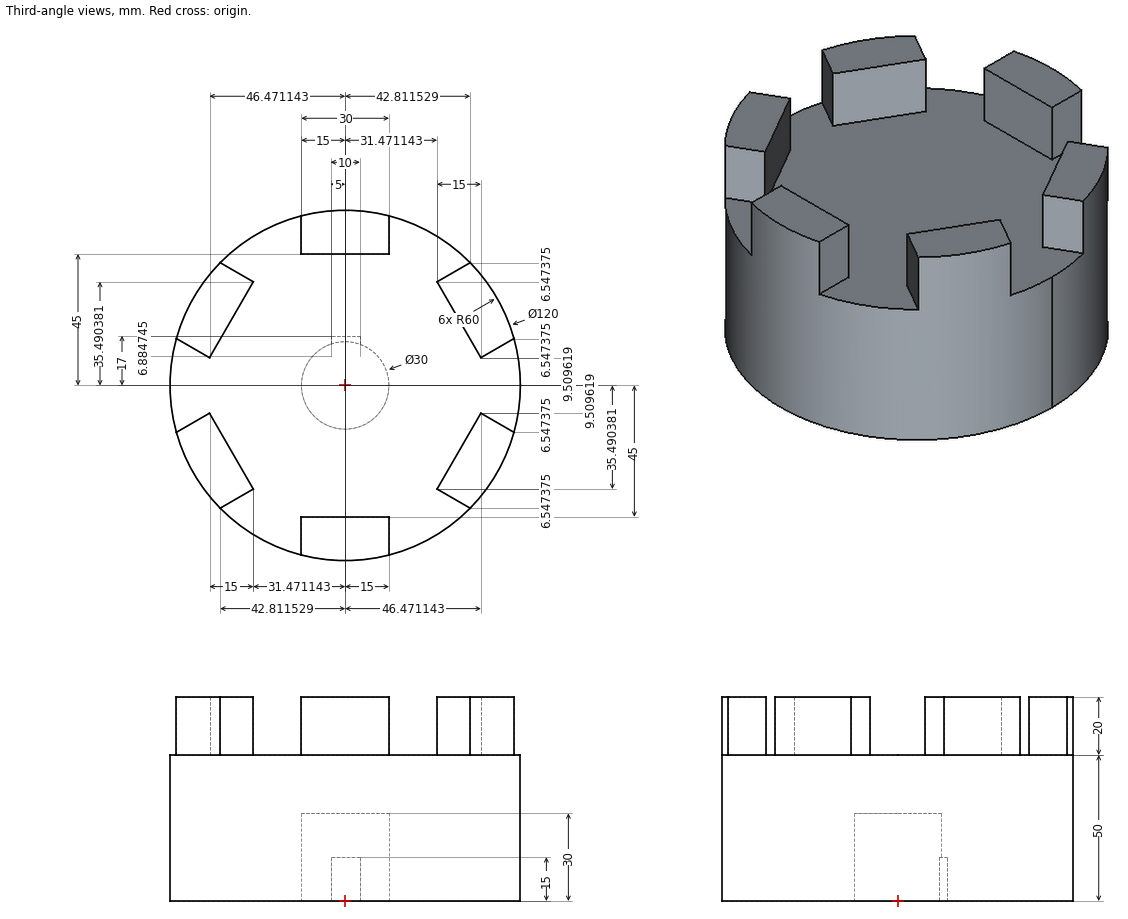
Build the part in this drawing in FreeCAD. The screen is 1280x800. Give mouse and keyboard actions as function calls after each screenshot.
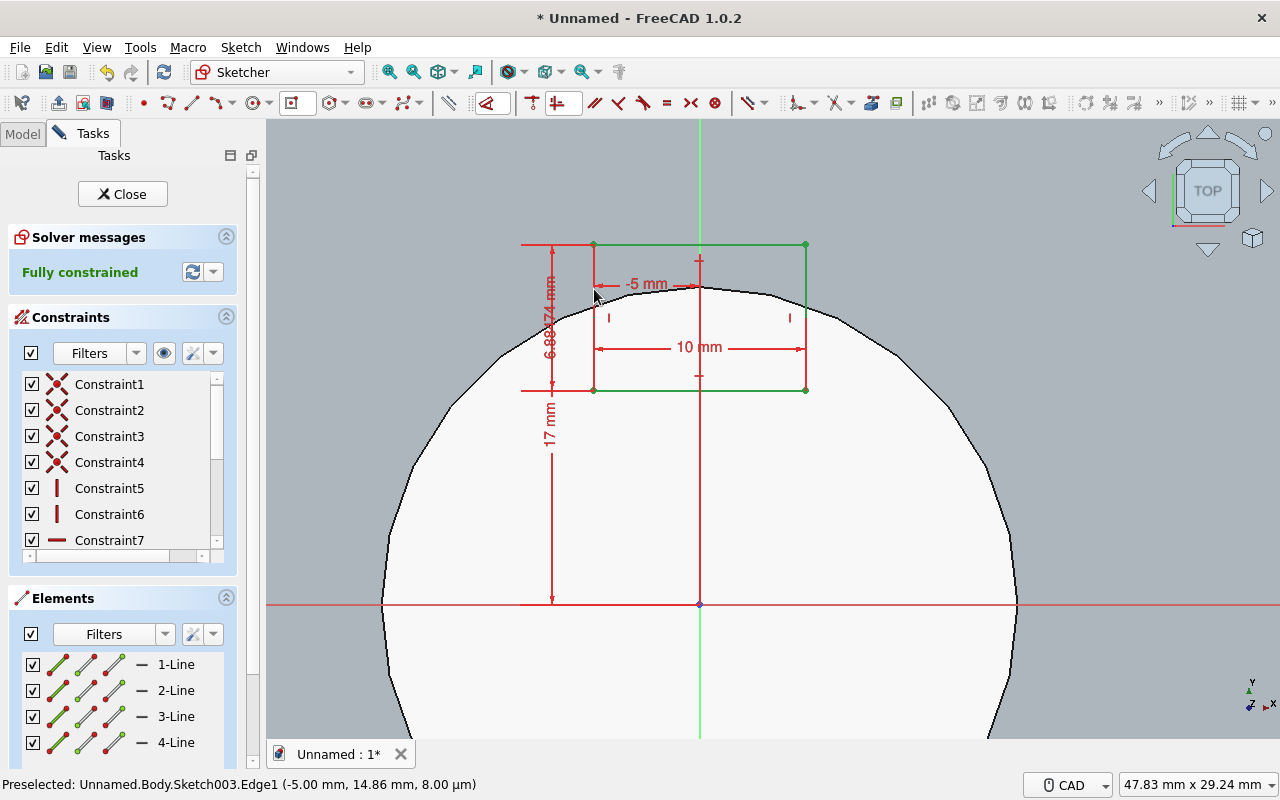
click(123, 194)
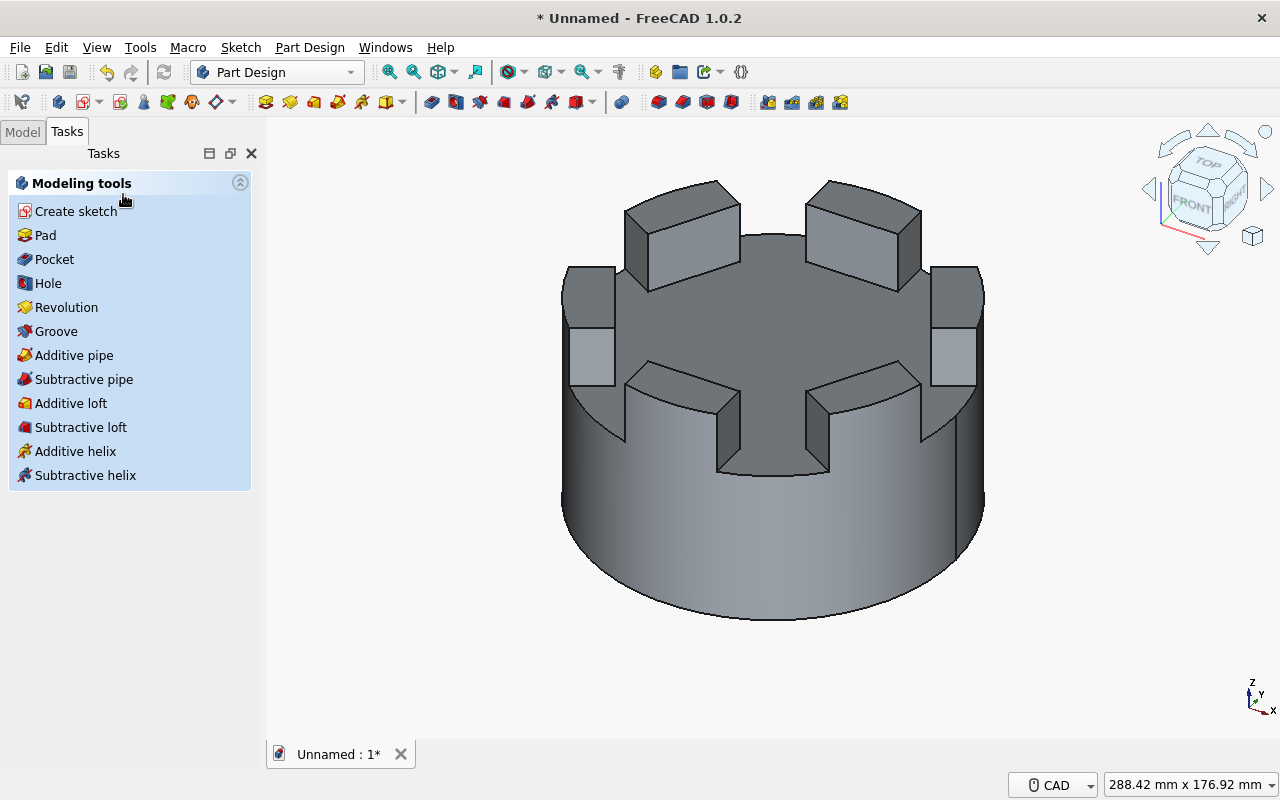
click(432, 102)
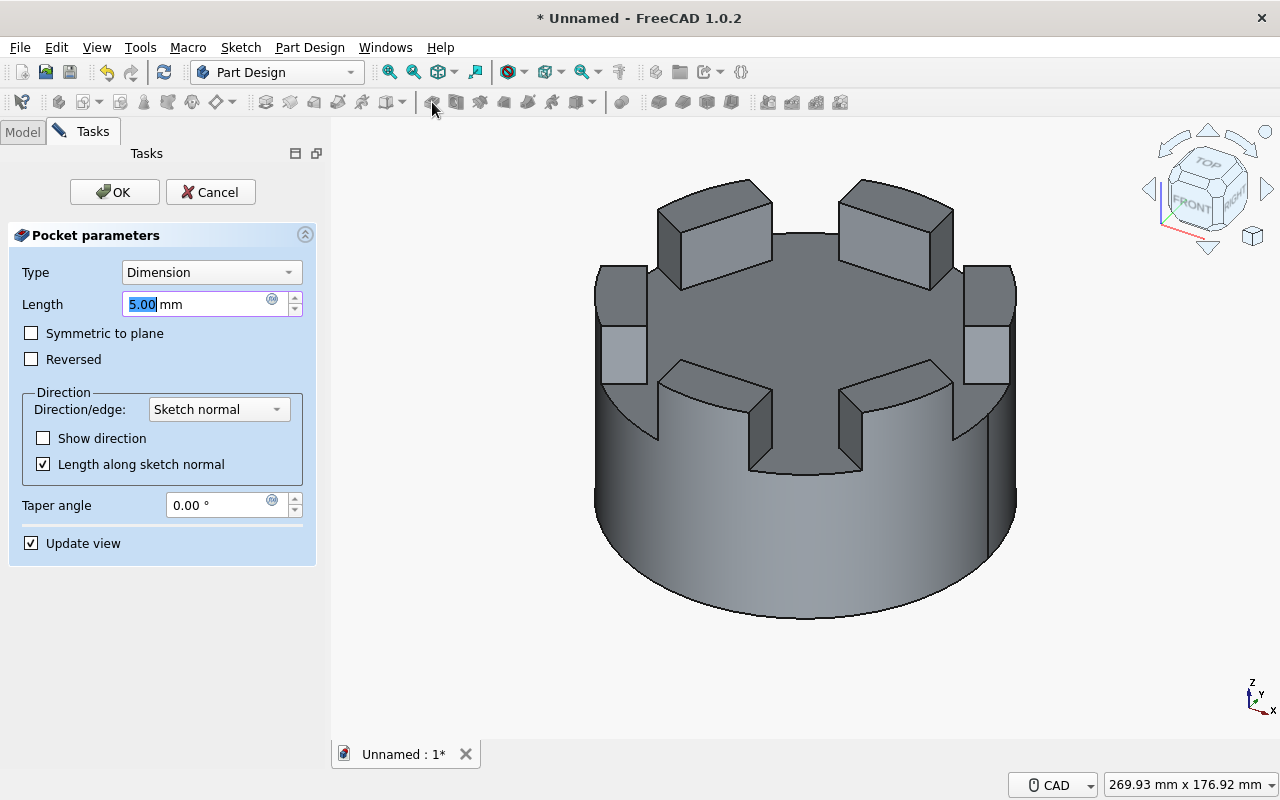
text(15)
key(Tab)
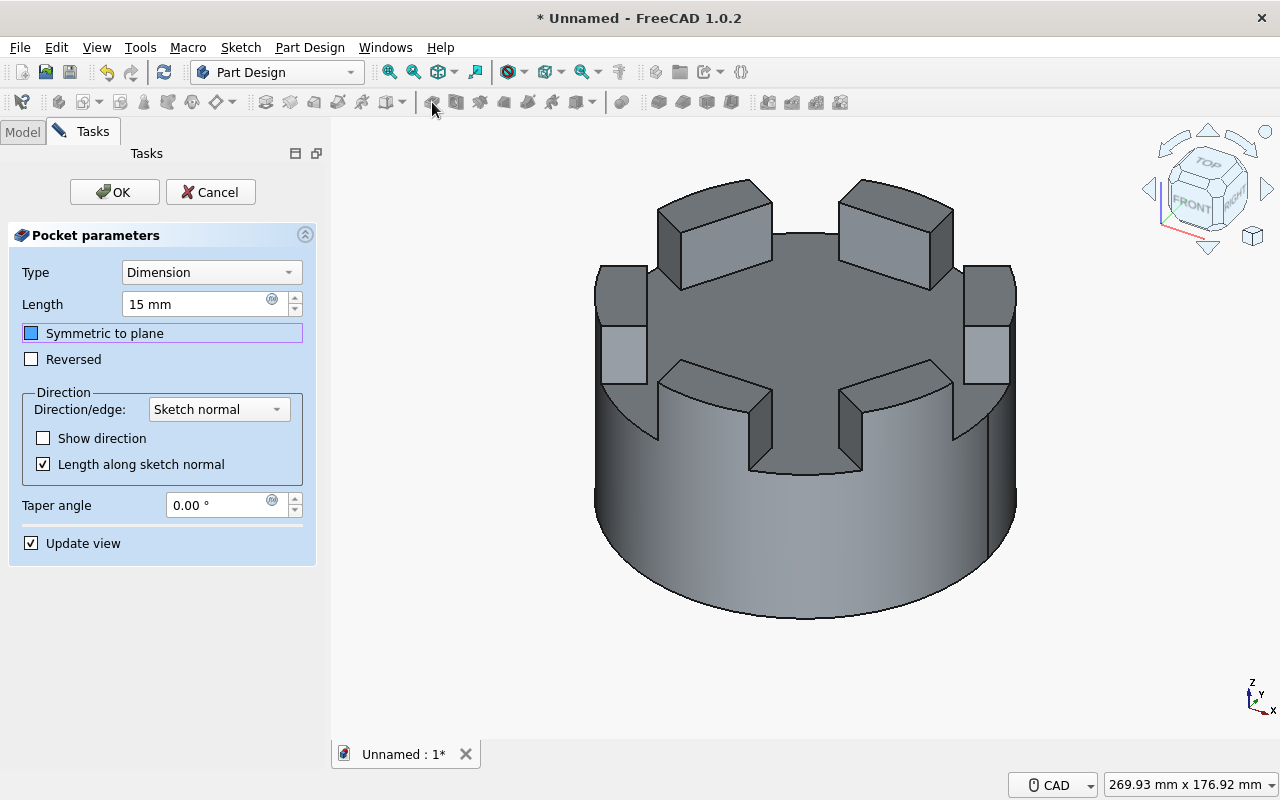
click(30, 359)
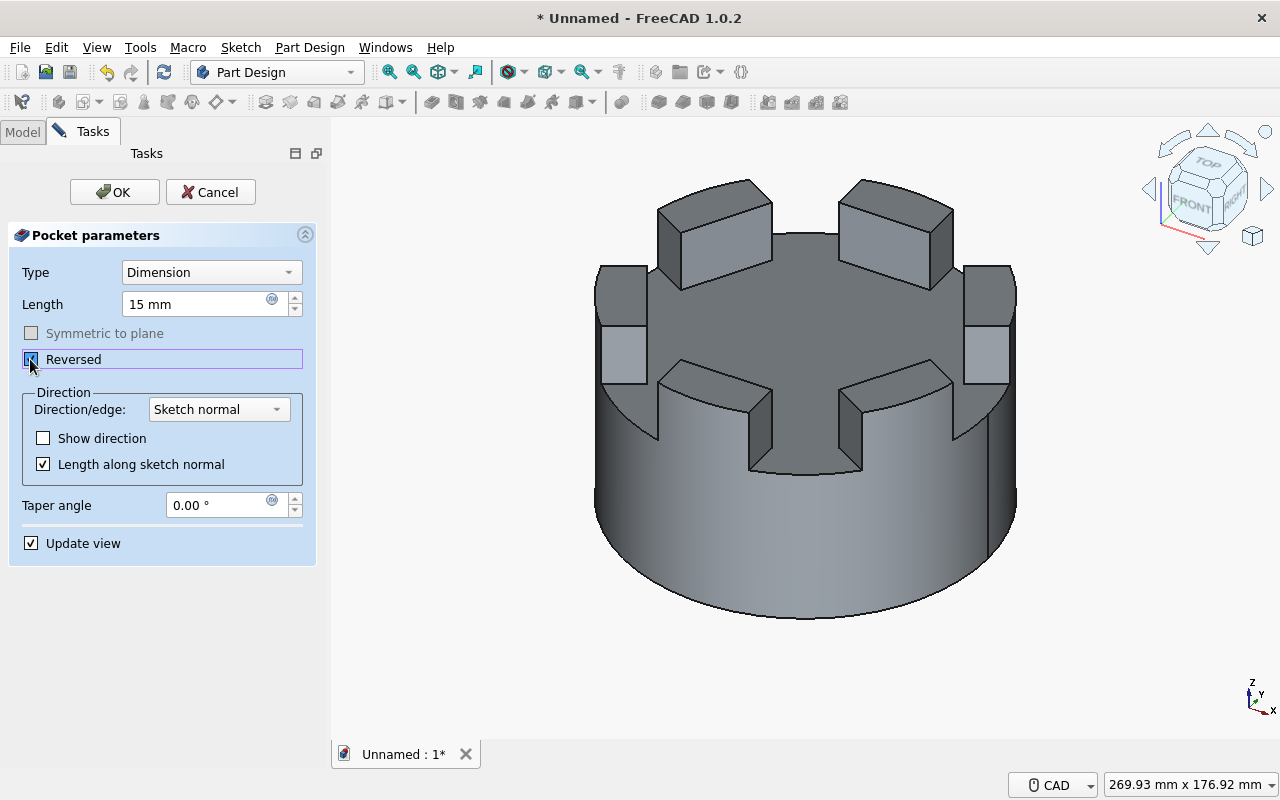
click(115, 192)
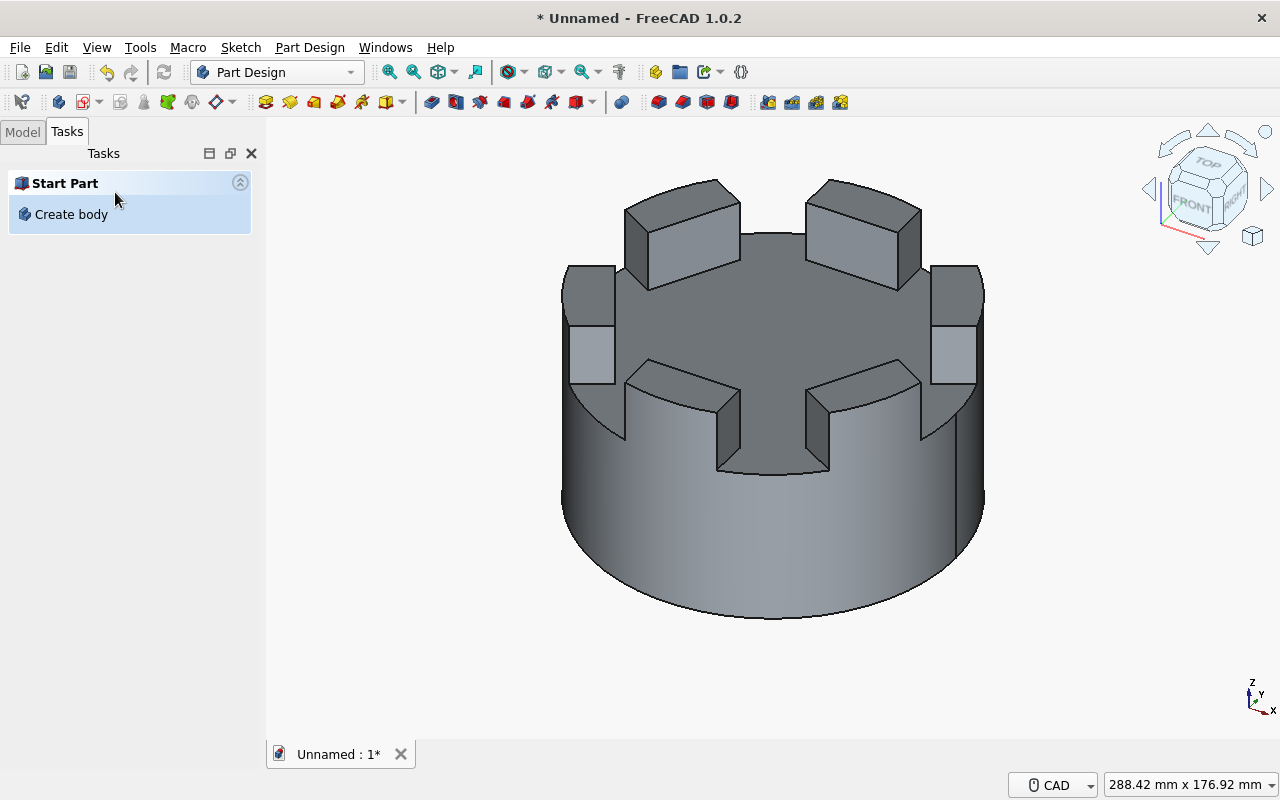
key(0)